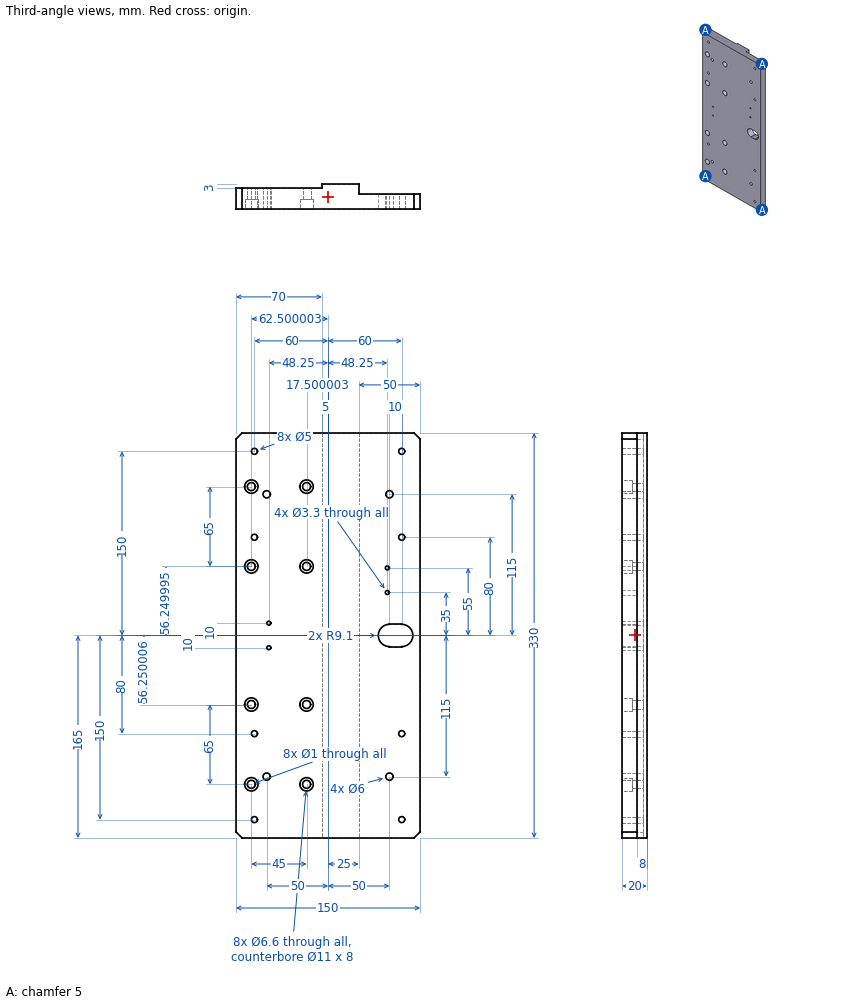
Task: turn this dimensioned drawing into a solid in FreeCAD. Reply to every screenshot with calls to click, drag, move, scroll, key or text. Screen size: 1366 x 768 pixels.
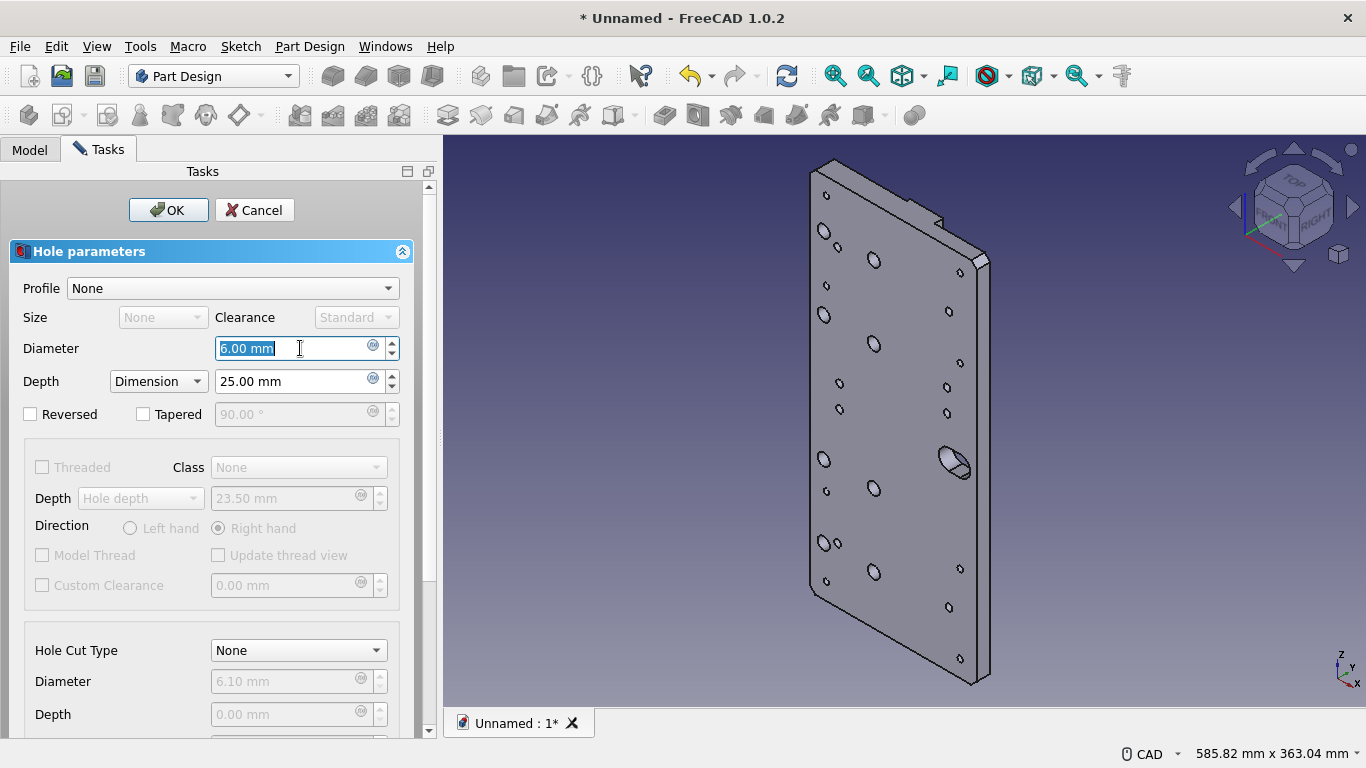
text(3.3)
key(Tab)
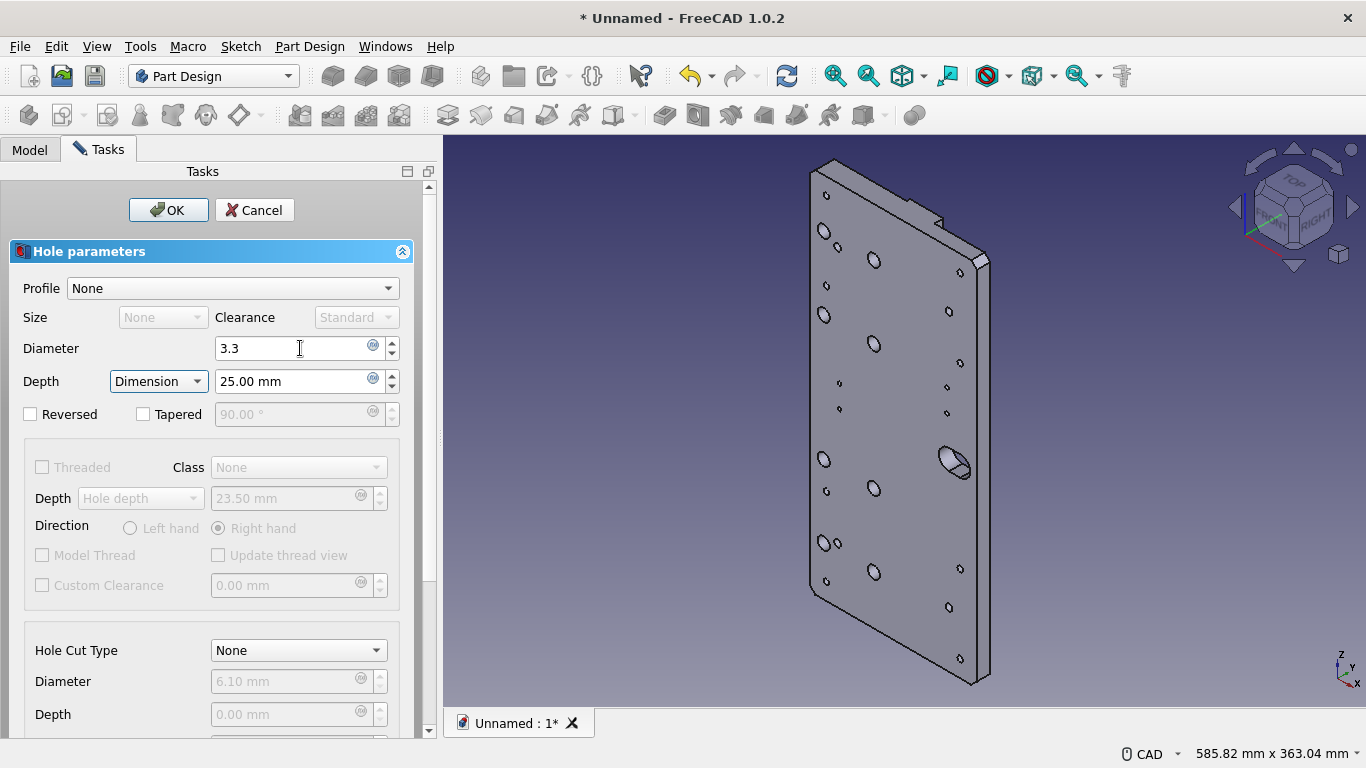
click(160, 382)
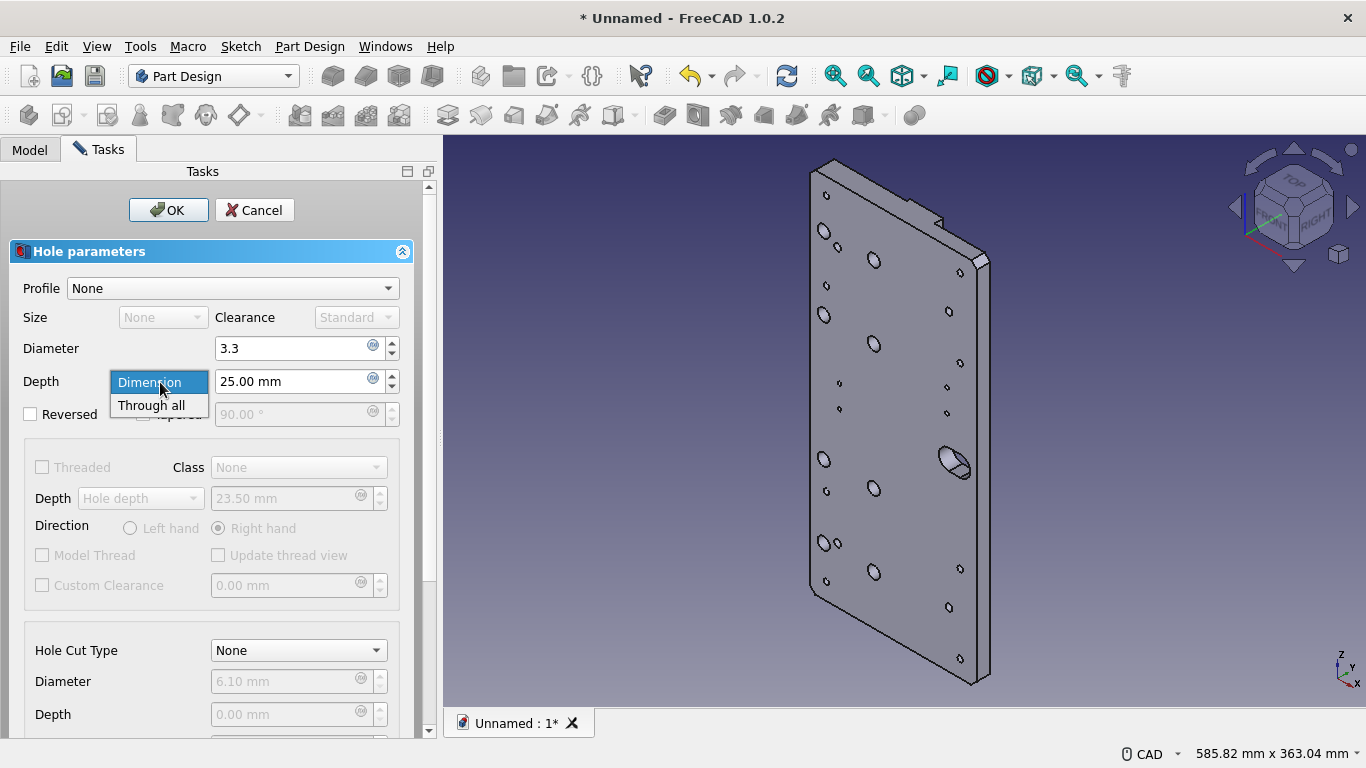
click(158, 406)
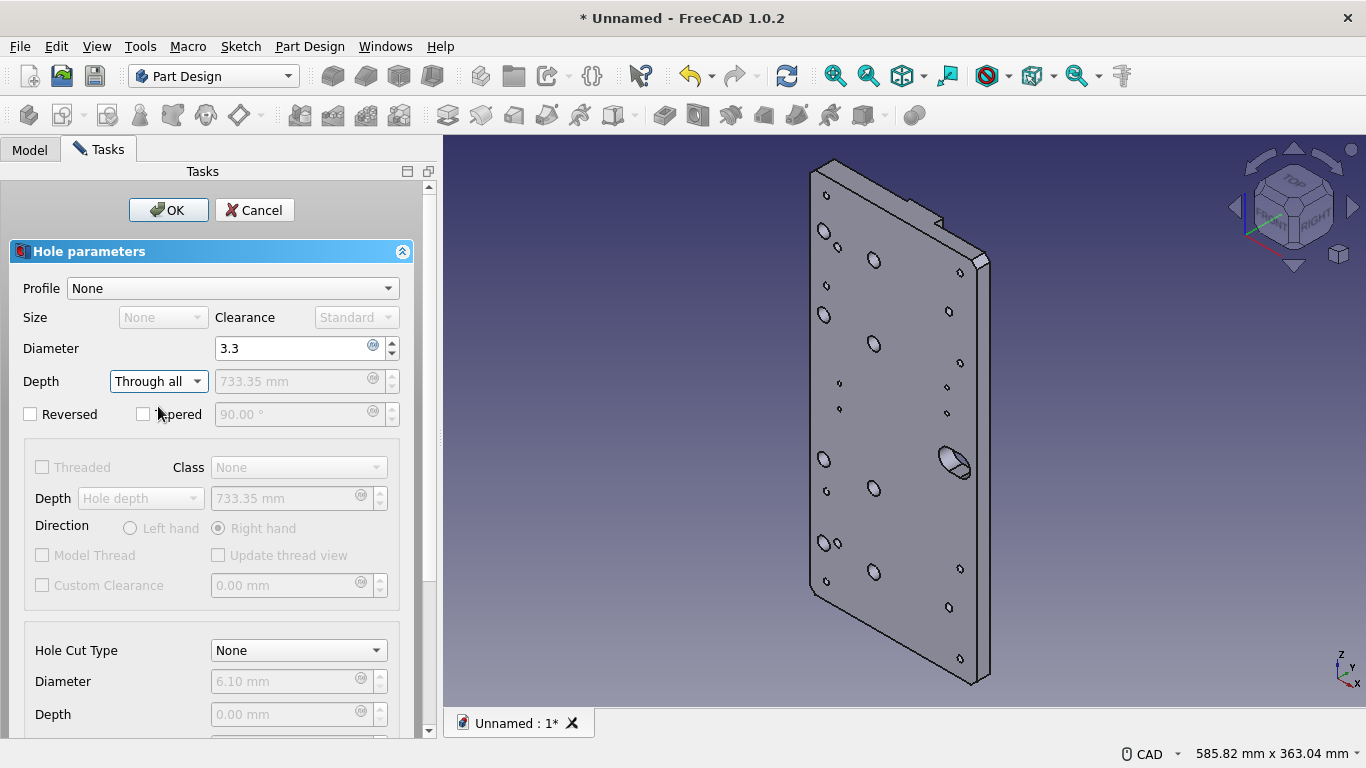
click(169, 210)